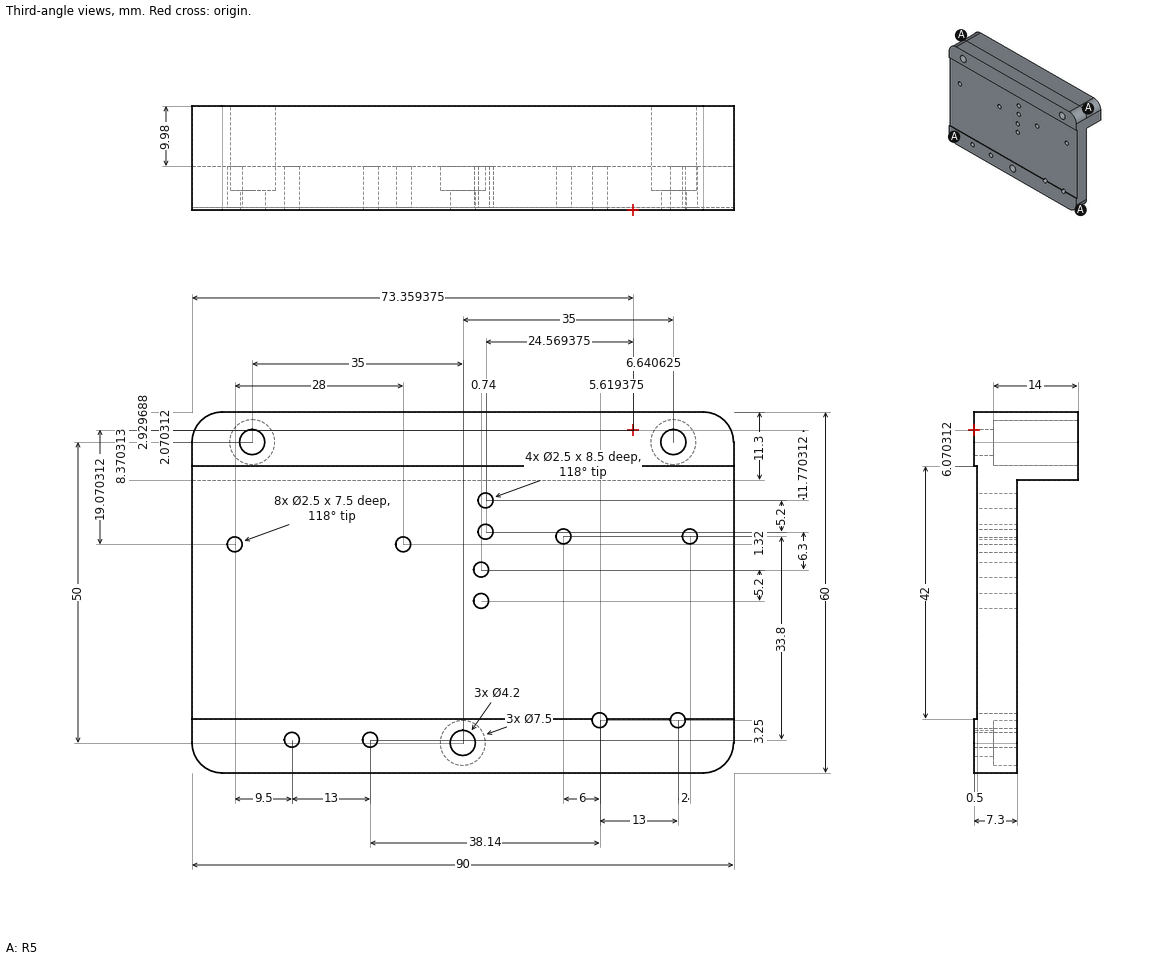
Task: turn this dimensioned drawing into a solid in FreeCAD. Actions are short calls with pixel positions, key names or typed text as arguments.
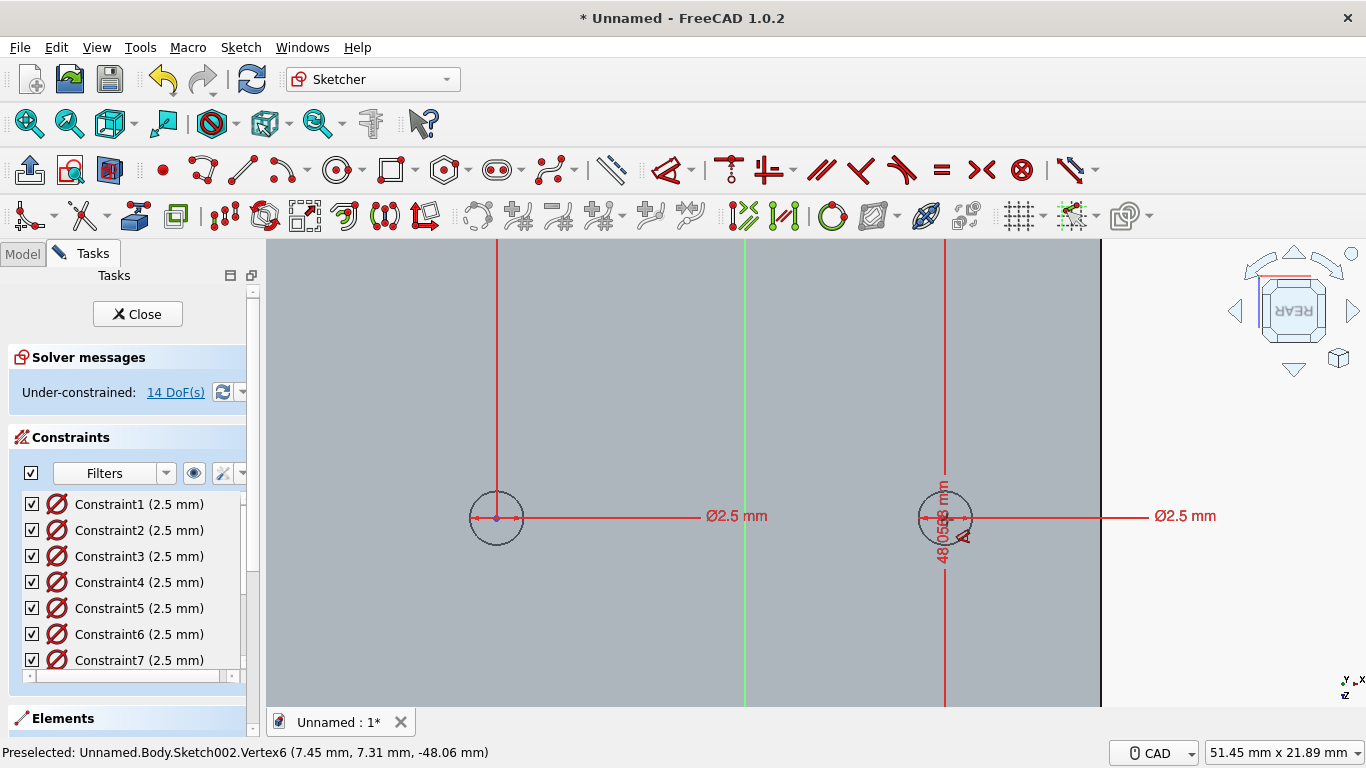
click(945, 518)
click(916, 552)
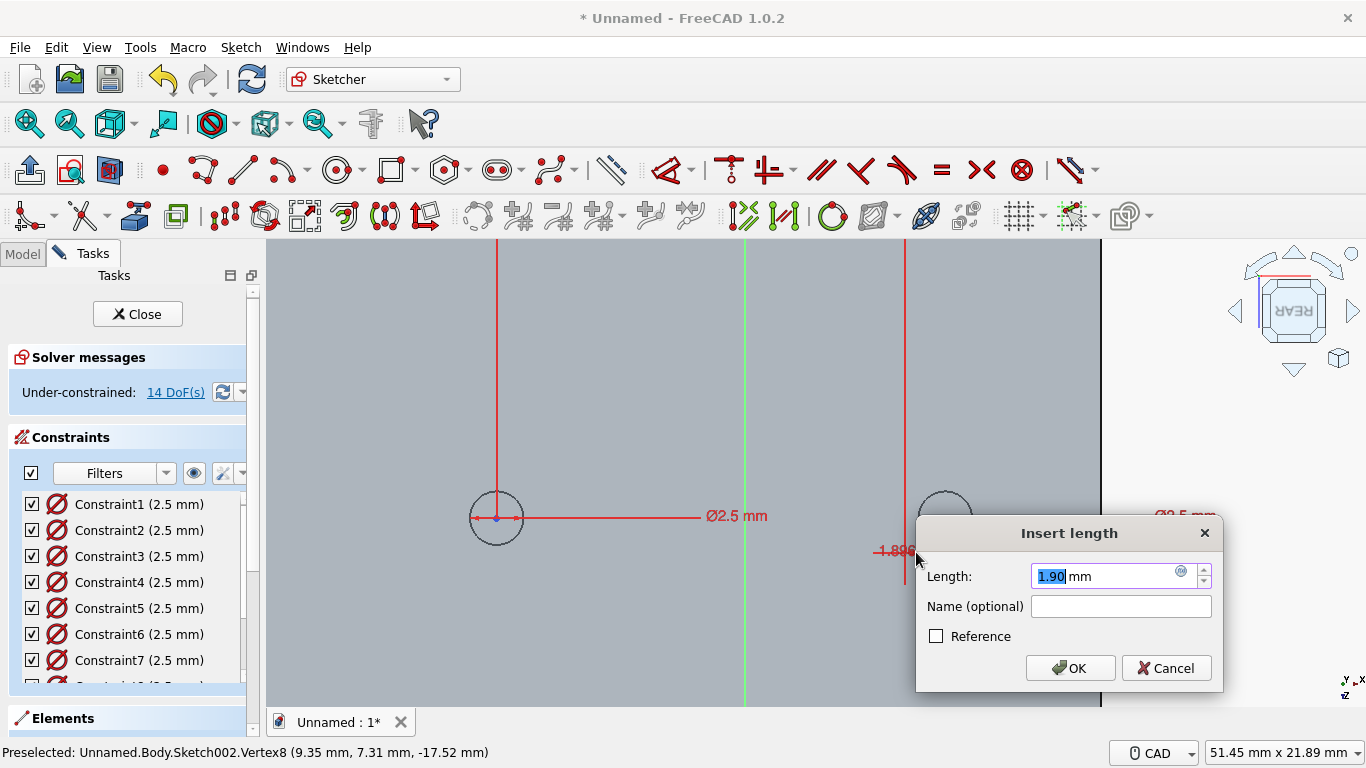
text(2)
key(Return)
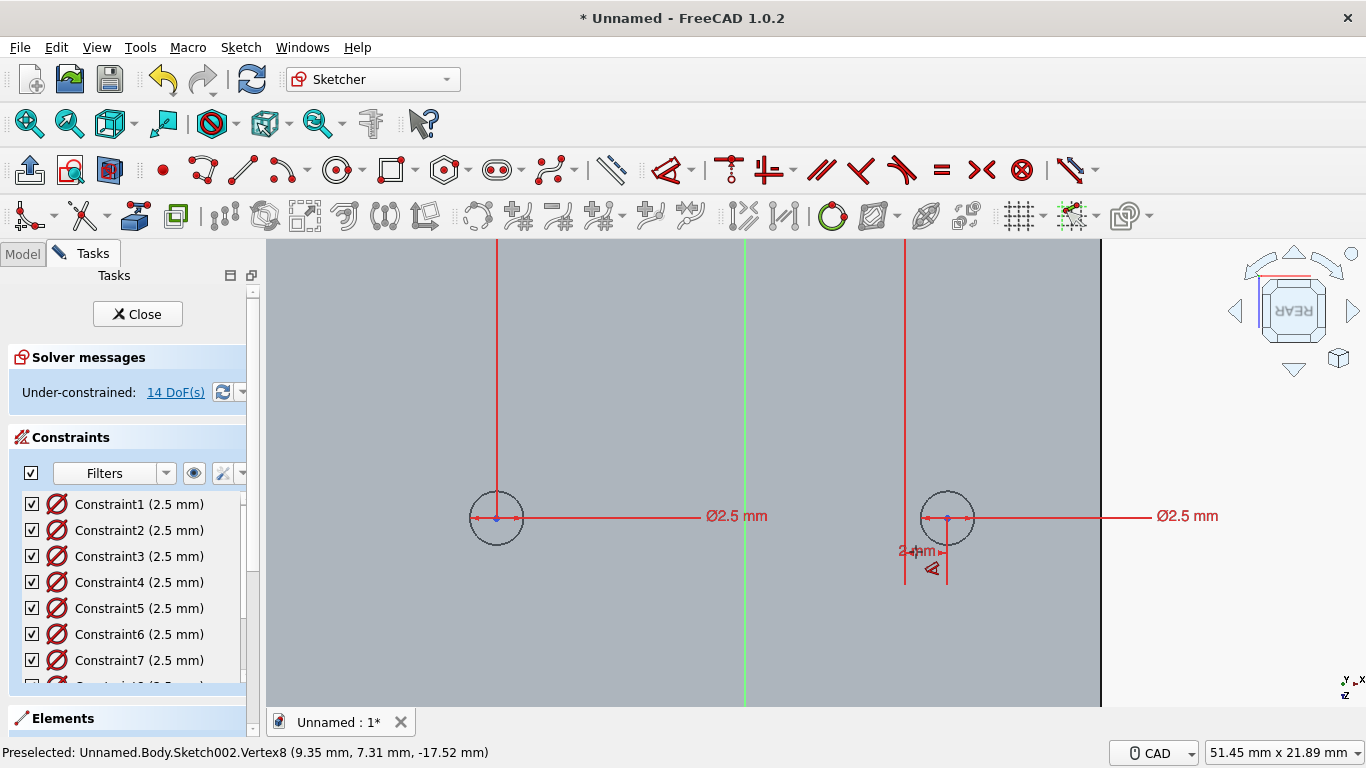
scroll(947, 520, down, 7)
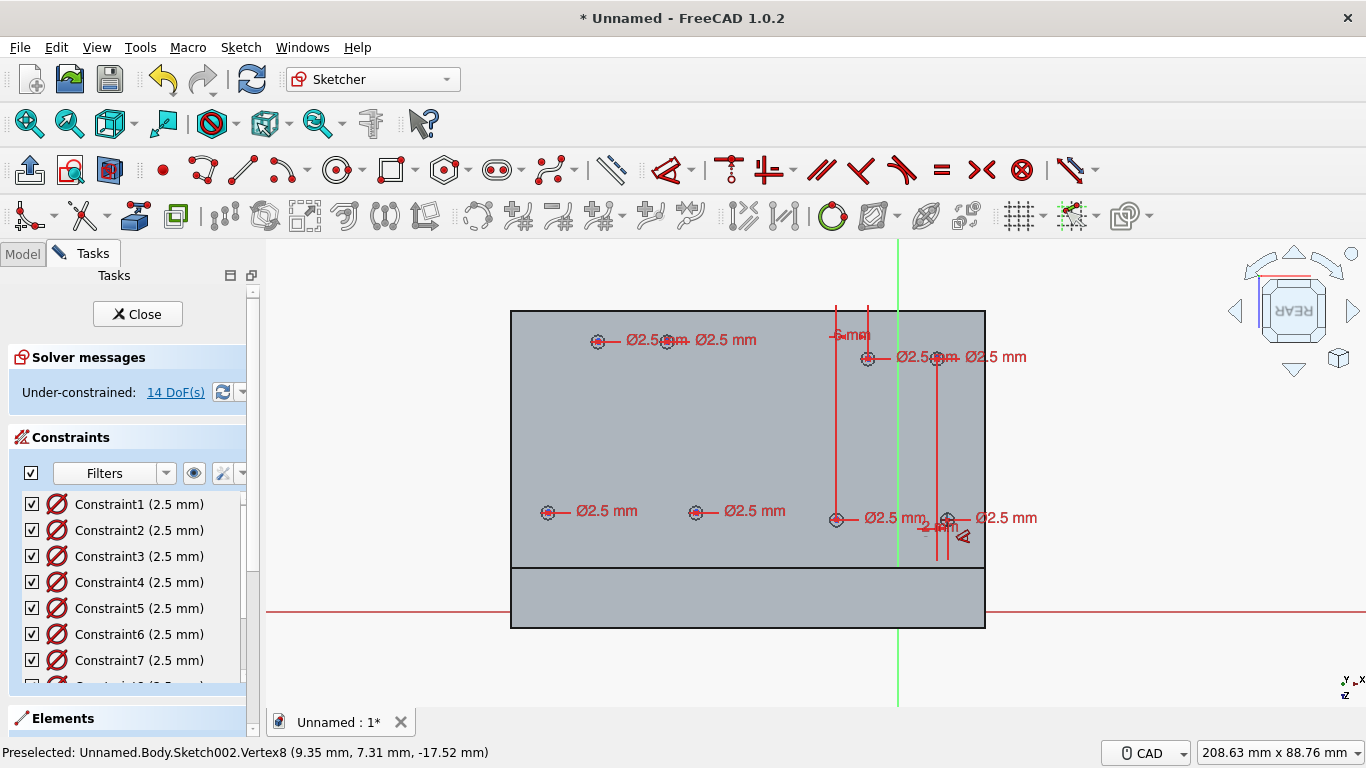
click(548, 513)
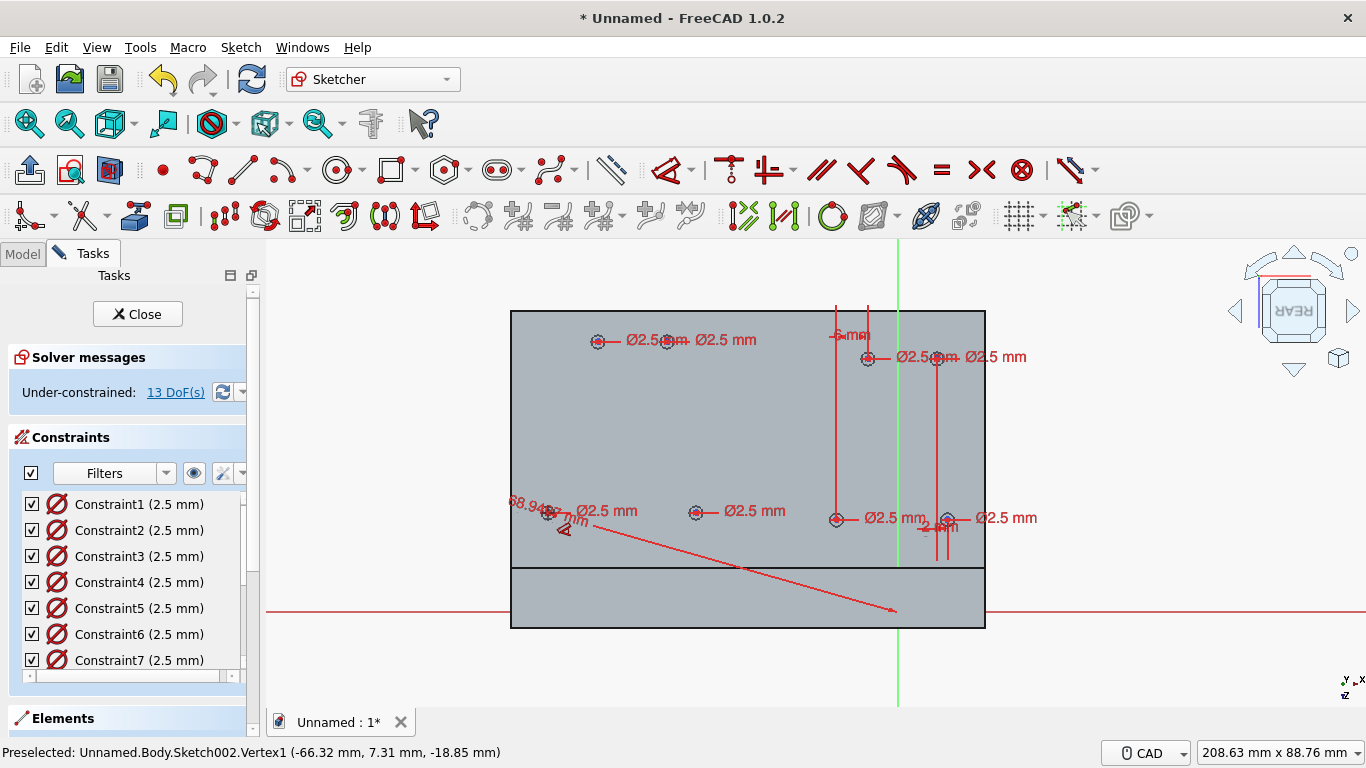
click(696, 513)
click(622, 547)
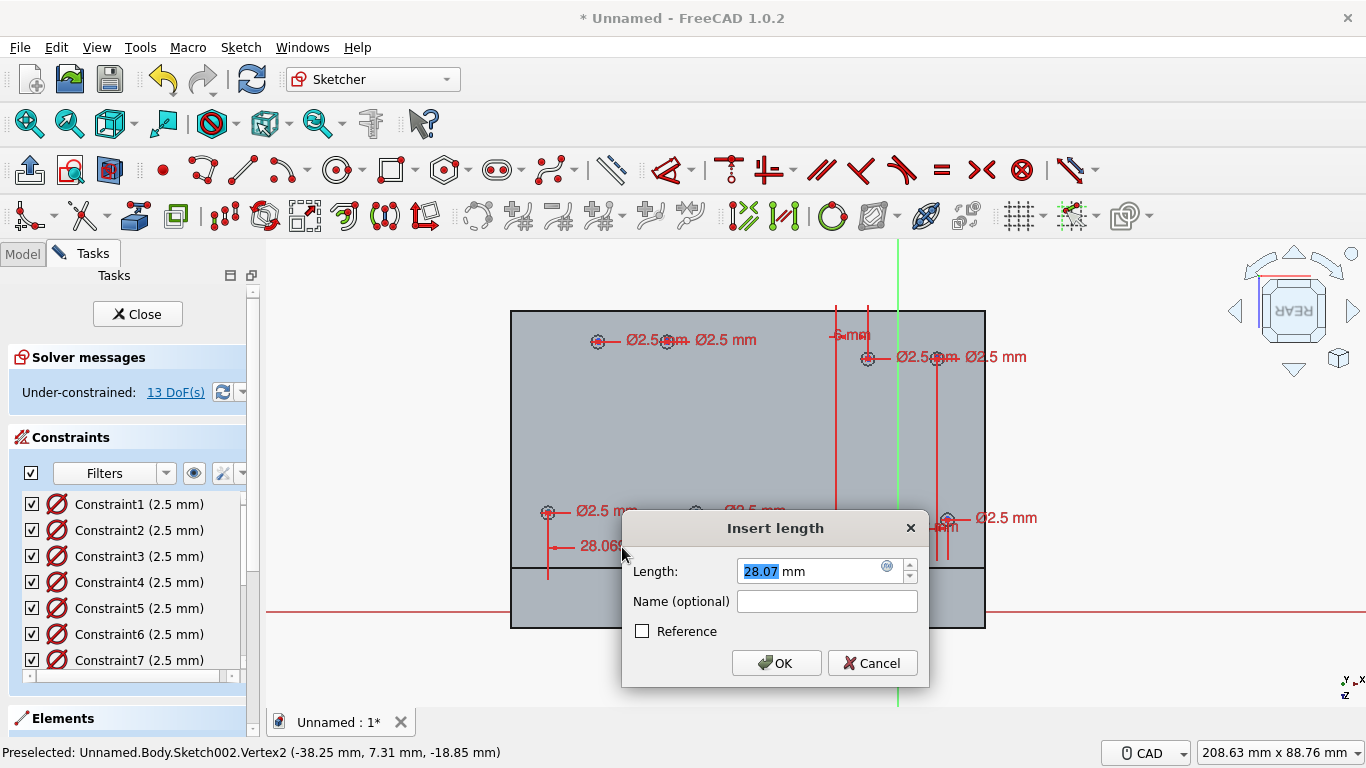
text(28)
key(Return)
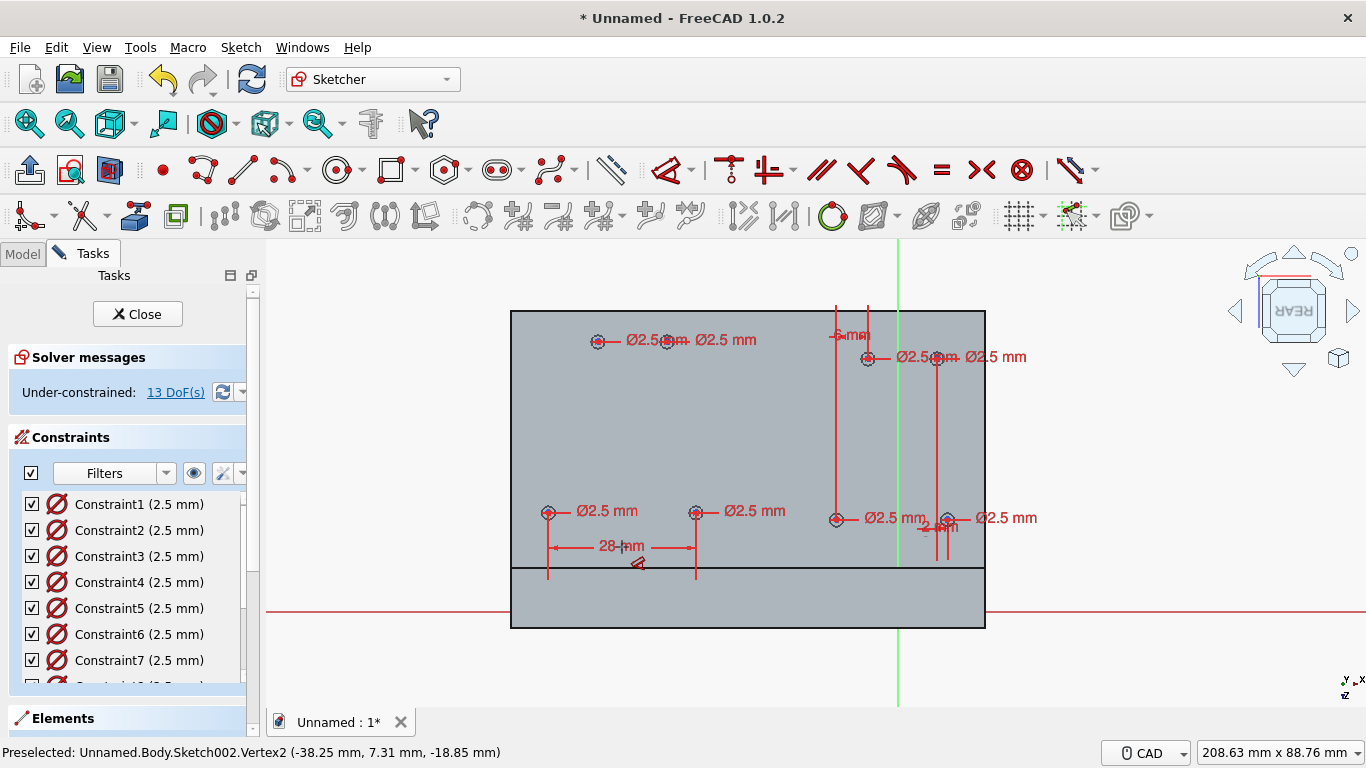
click(598, 342)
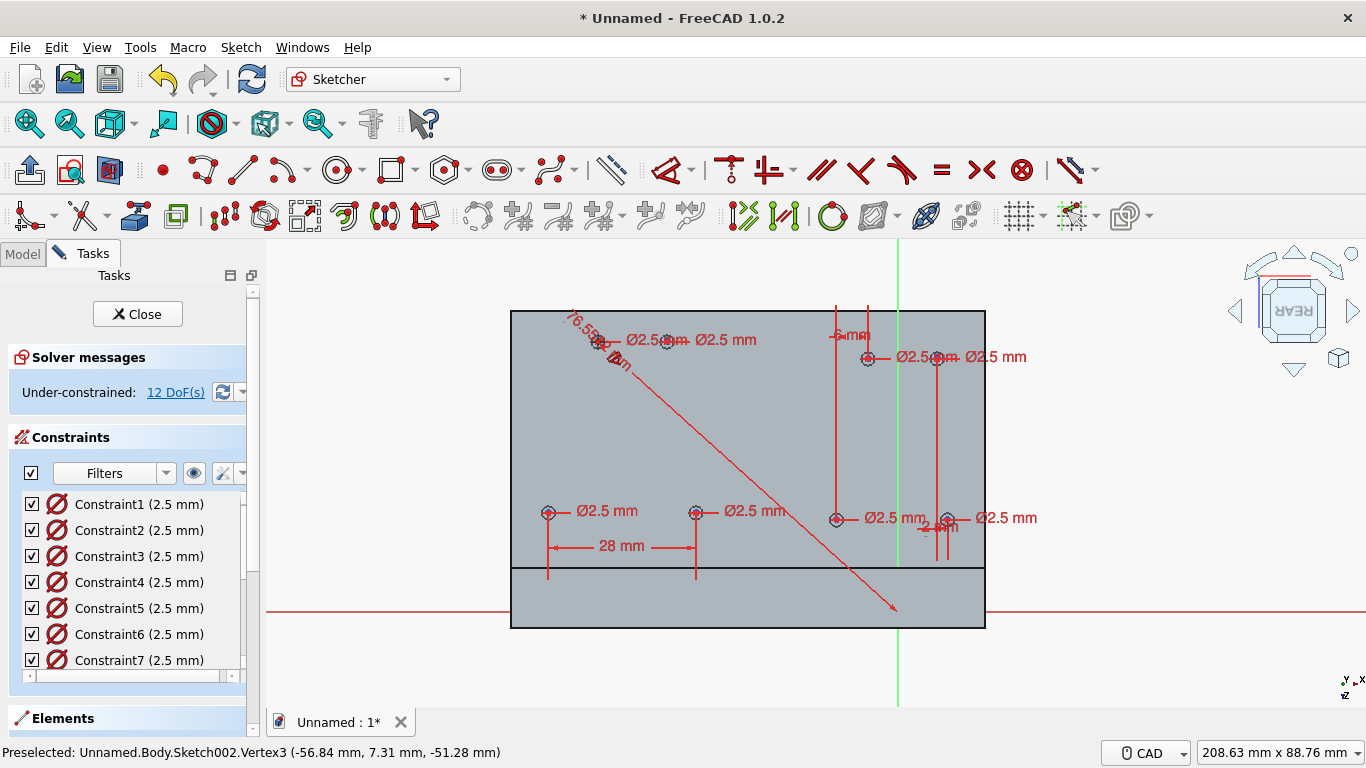
click(667, 342)
click(633, 308)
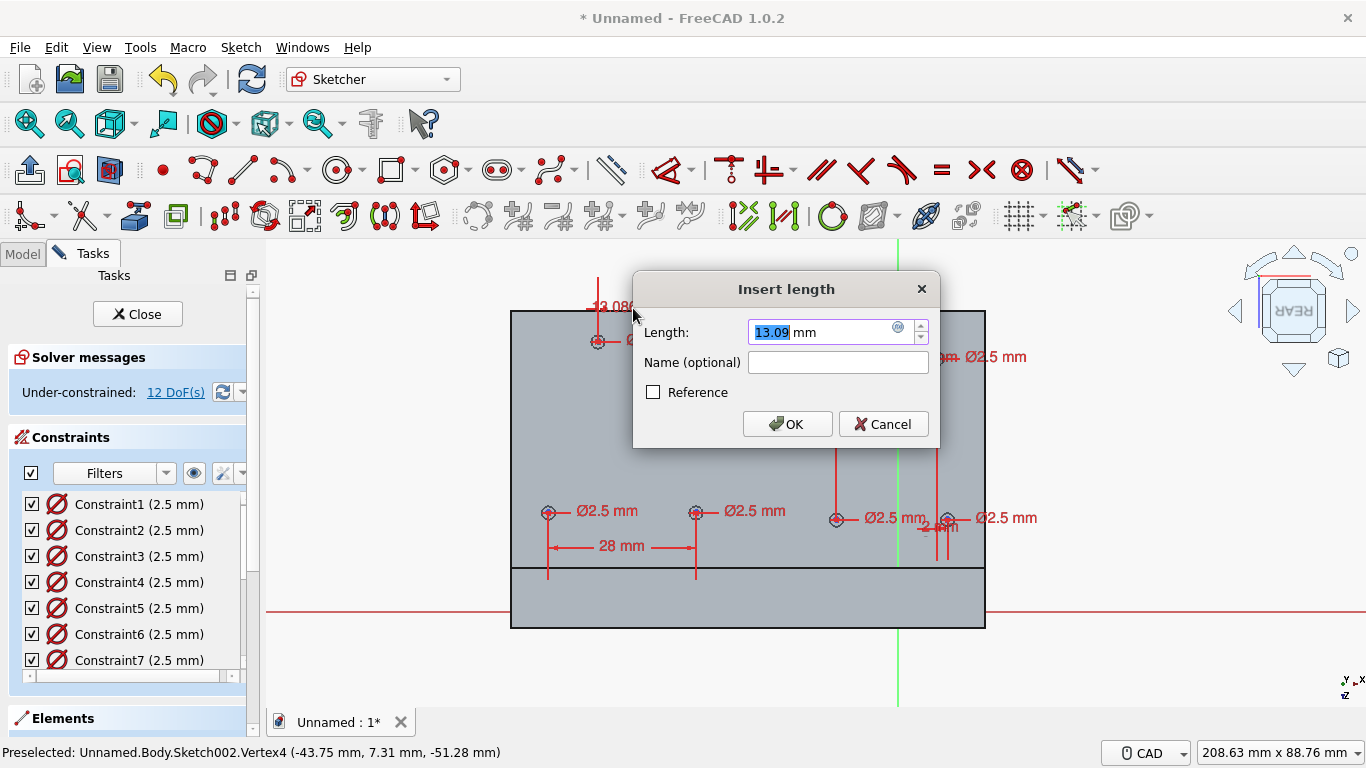
text(13)
key(Return)